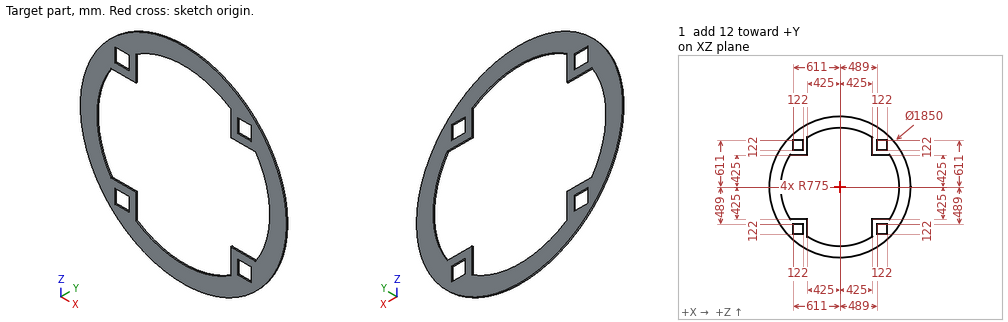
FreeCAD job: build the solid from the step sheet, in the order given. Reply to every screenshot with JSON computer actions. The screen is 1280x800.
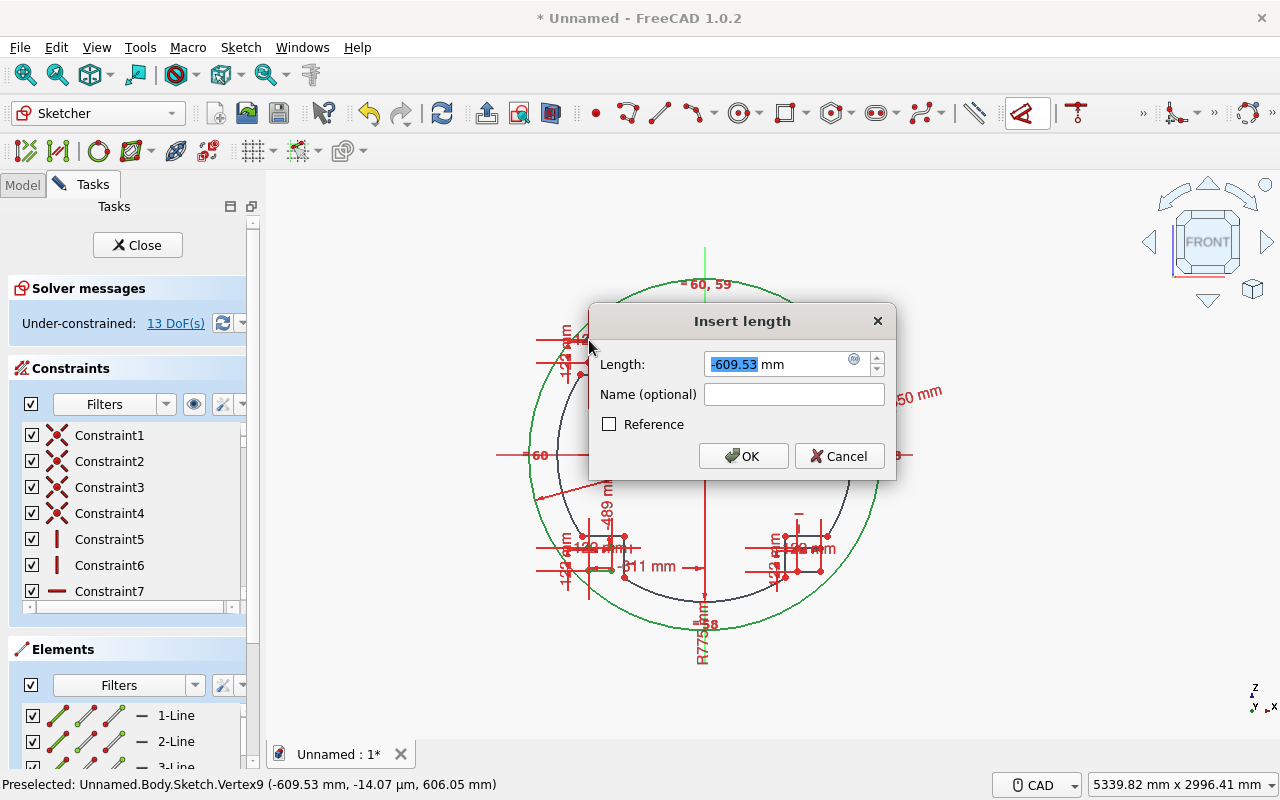
{"action": "type", "text": "-611"}
{"action": "key", "text": "Return"}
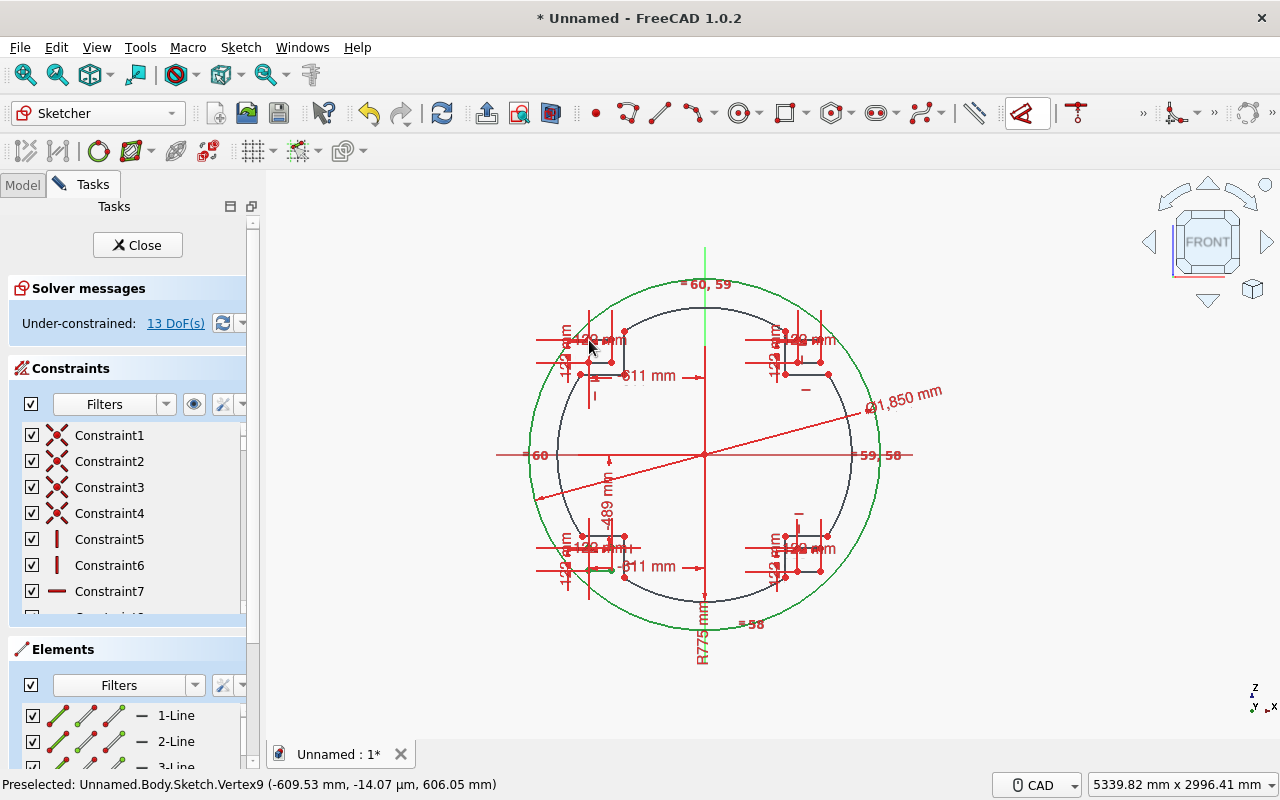
{"action": "left_click", "coordinate": [589, 340]}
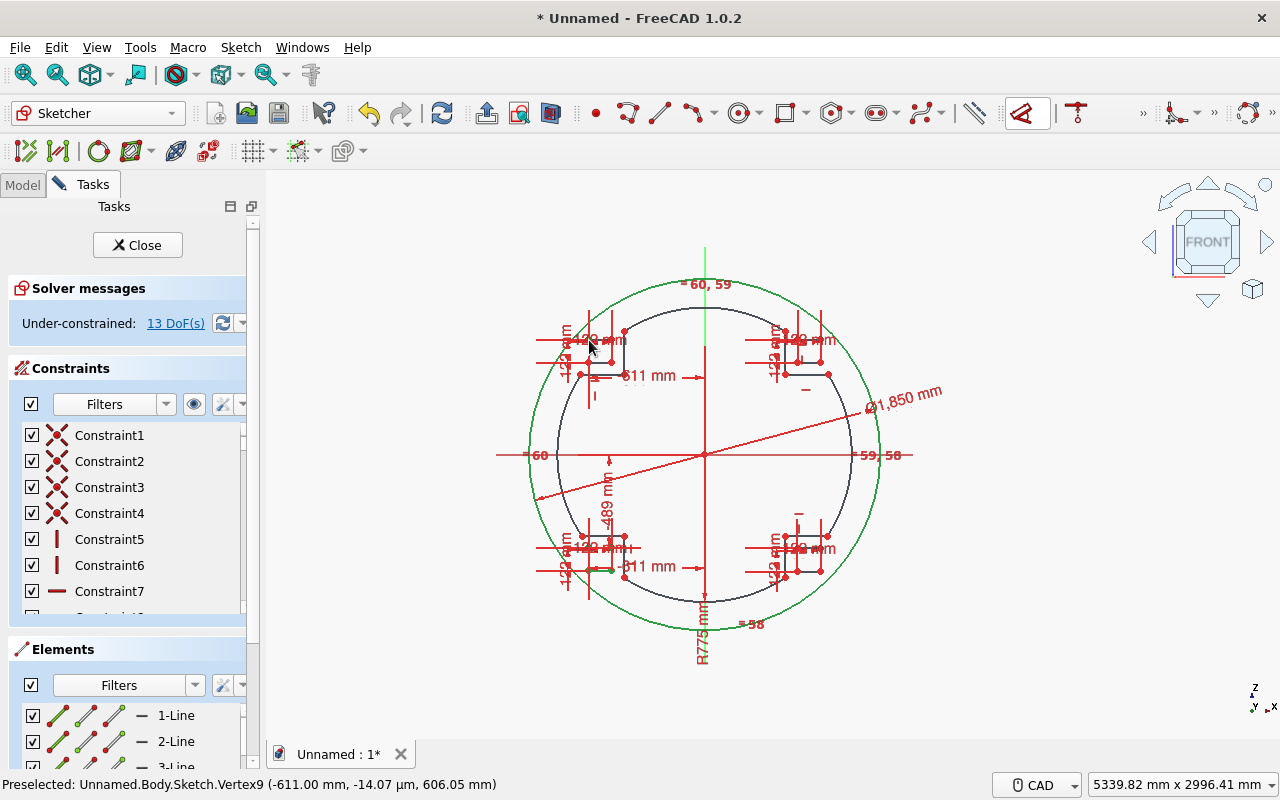
{"action": "key", "text": "i"}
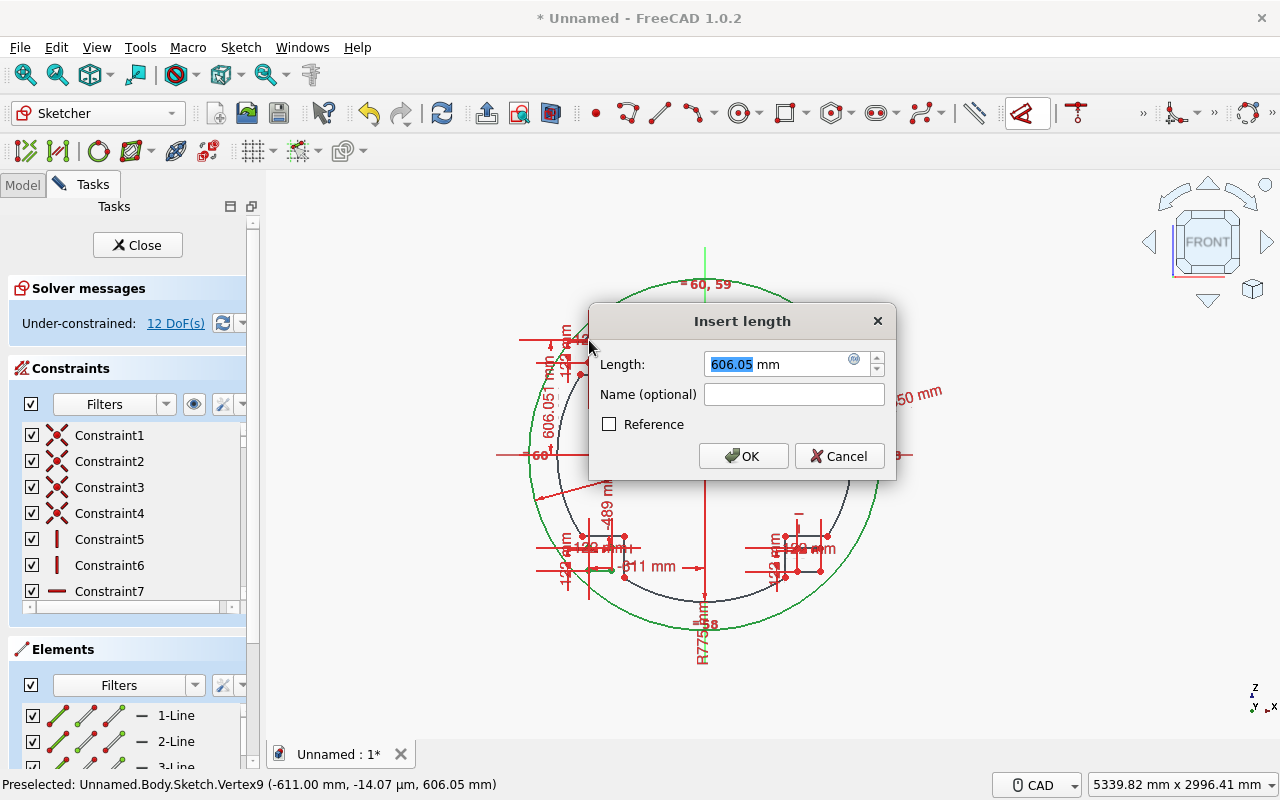
{"action": "type", "text": "611"}
{"action": "key", "text": "Return"}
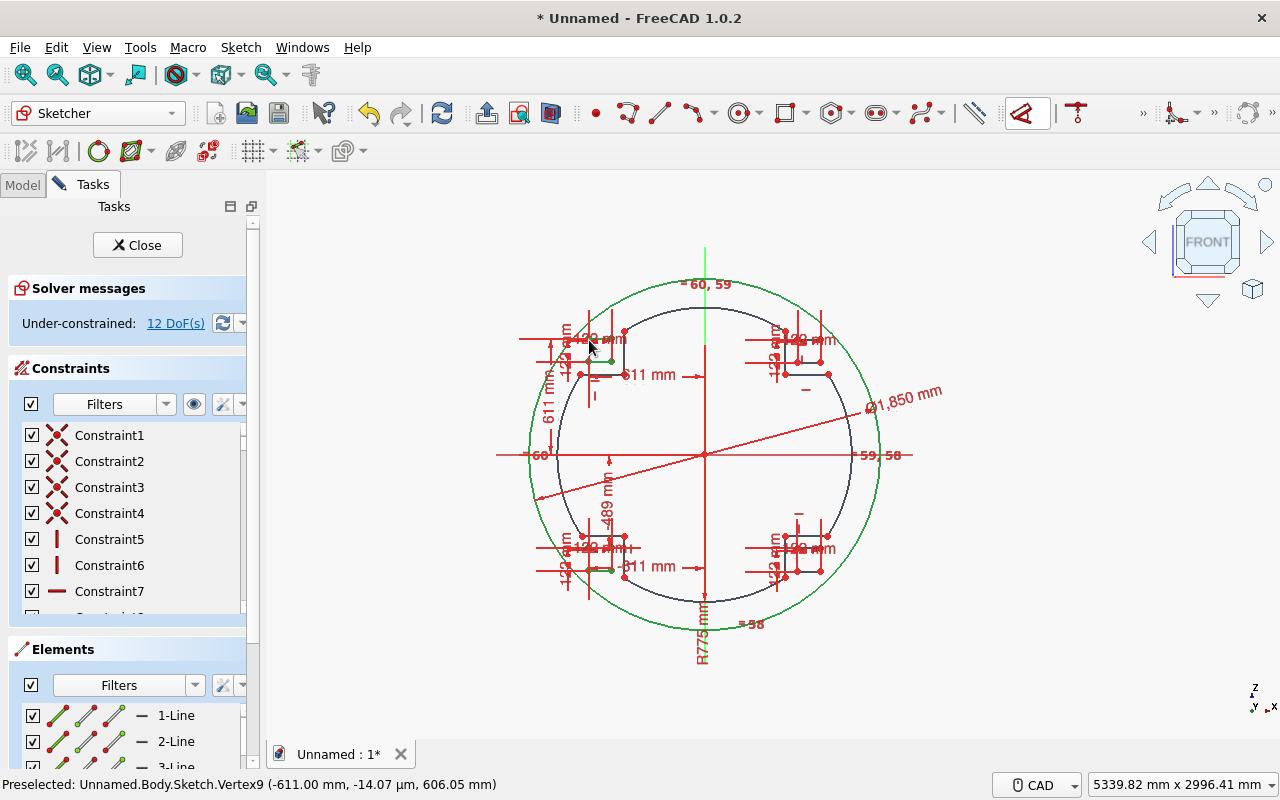
{"action": "left_click", "coordinate": [797, 548]}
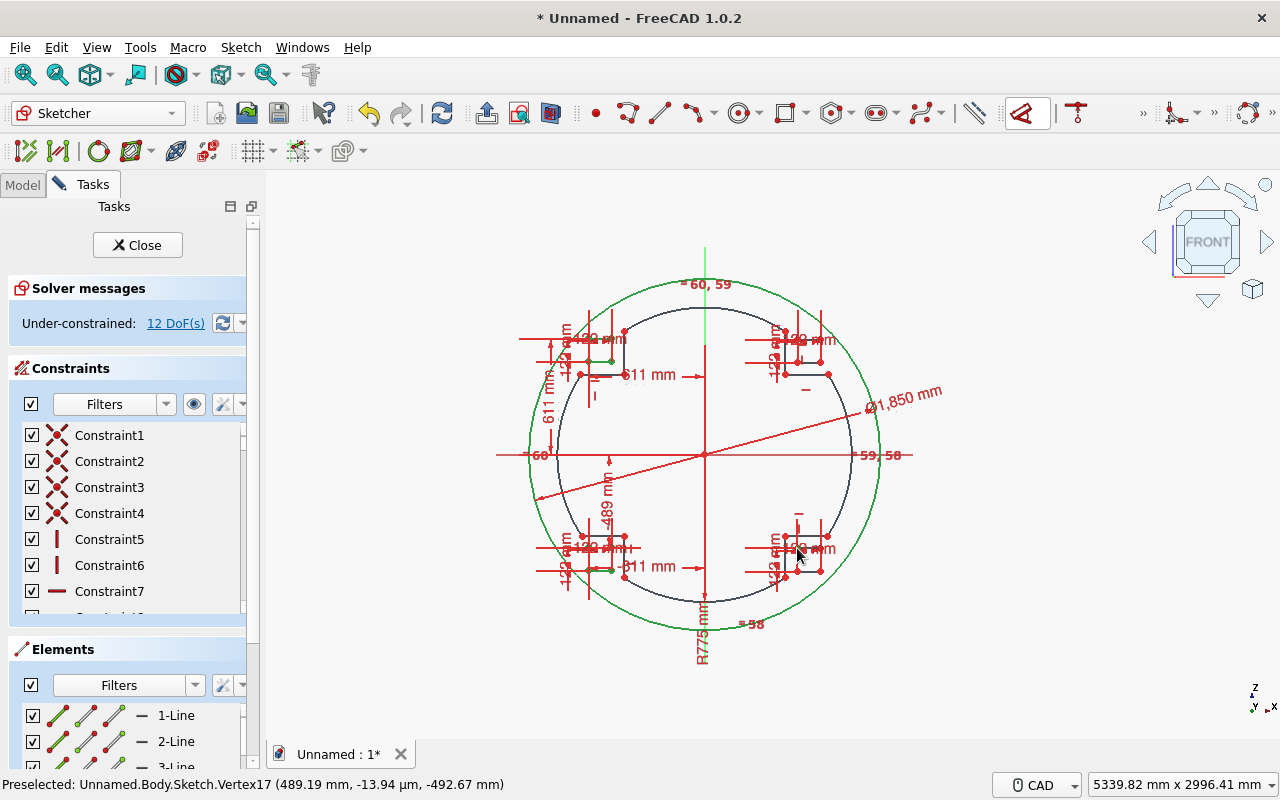
{"action": "key", "text": "l"}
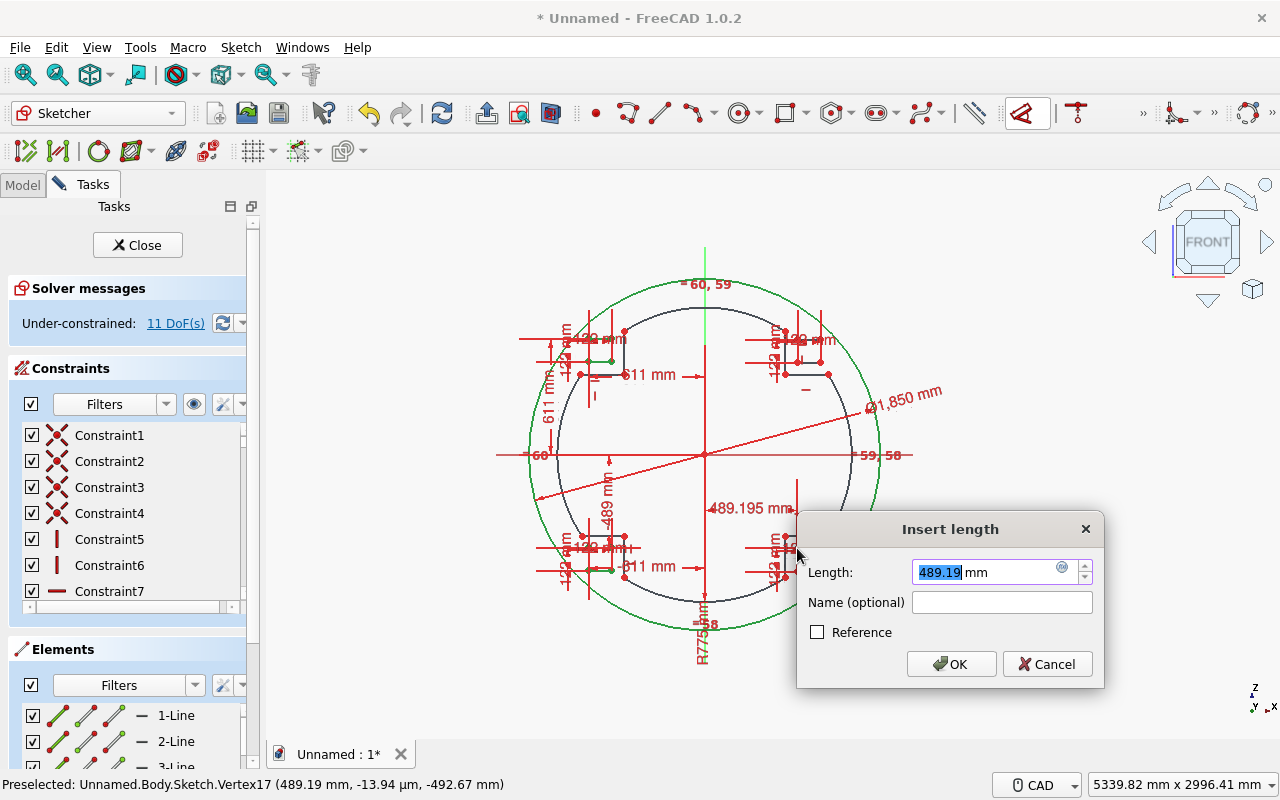
{"action": "type", "text": "489"}
{"action": "key", "text": "Return"}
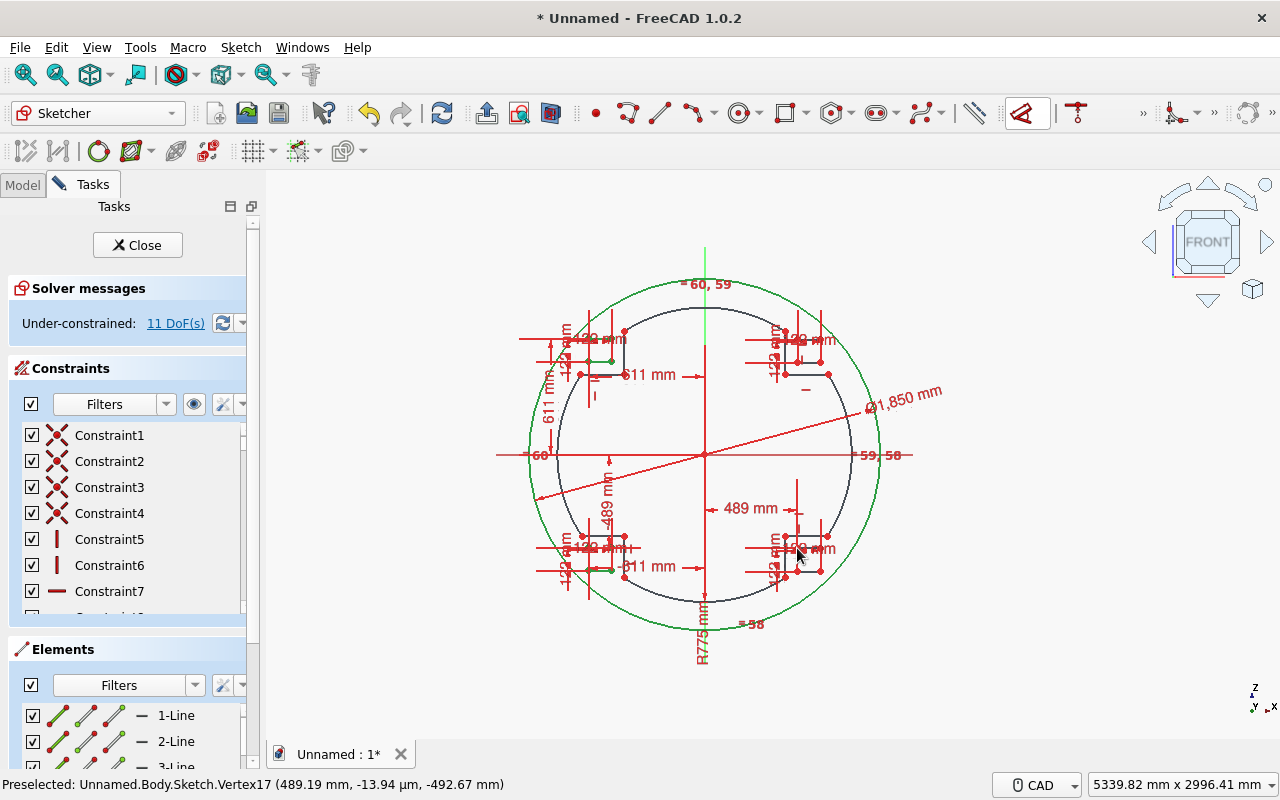
{"action": "left_click", "coordinate": [797, 548]}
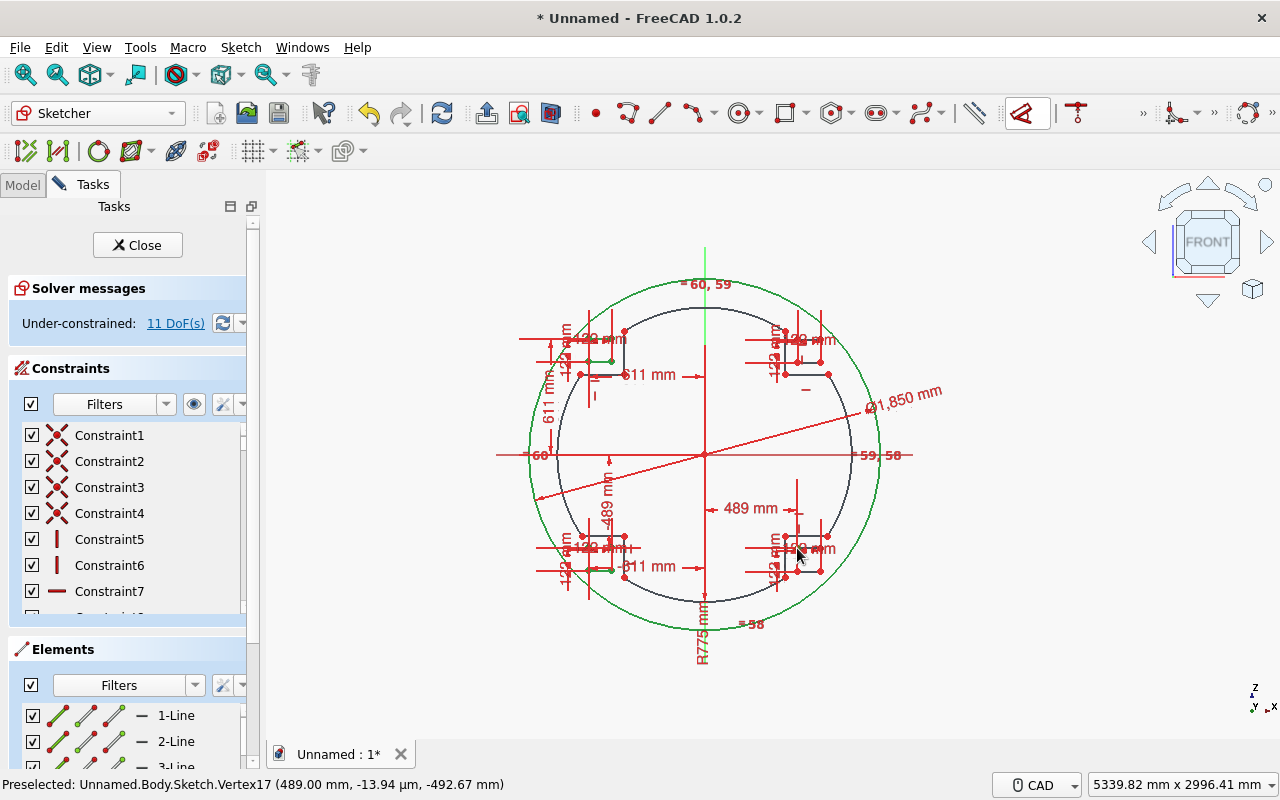
{"action": "key", "text": "i"}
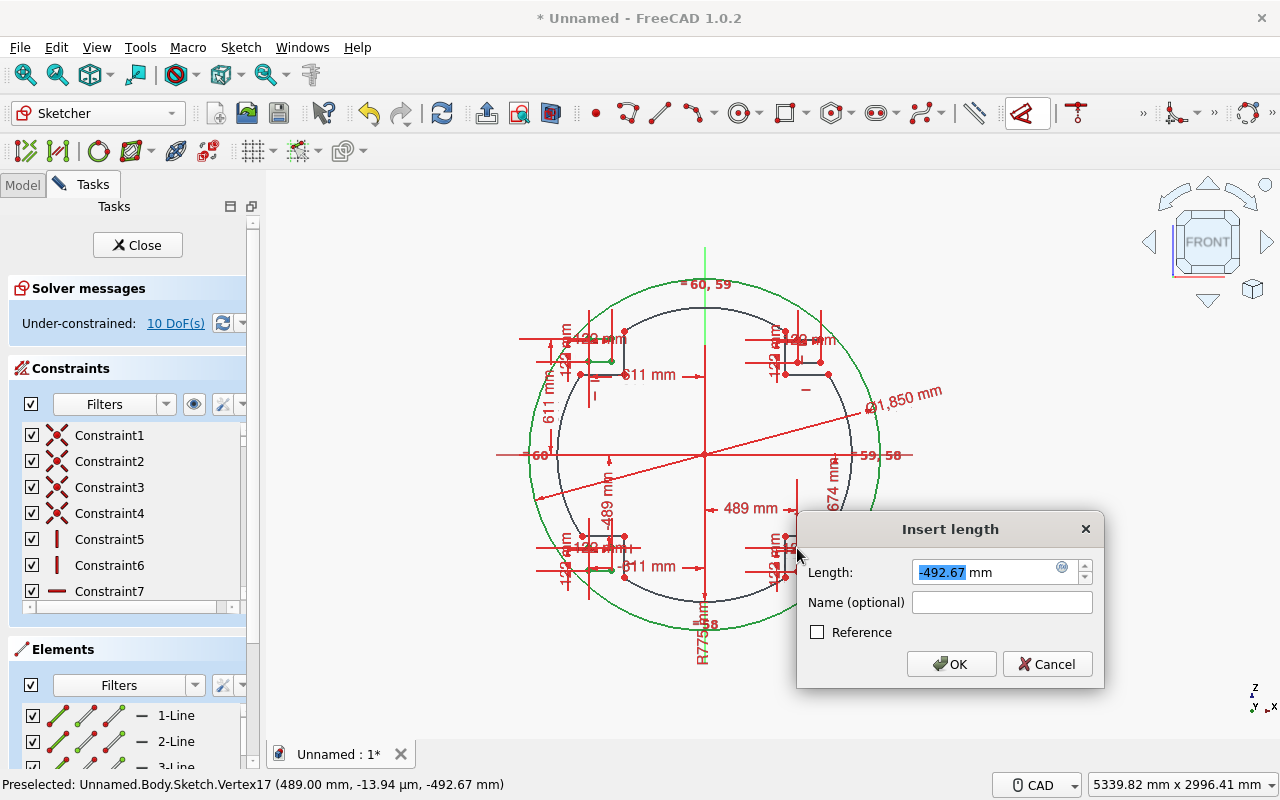
{"action": "type", "text": "-489"}
{"action": "key", "text": "Return"}